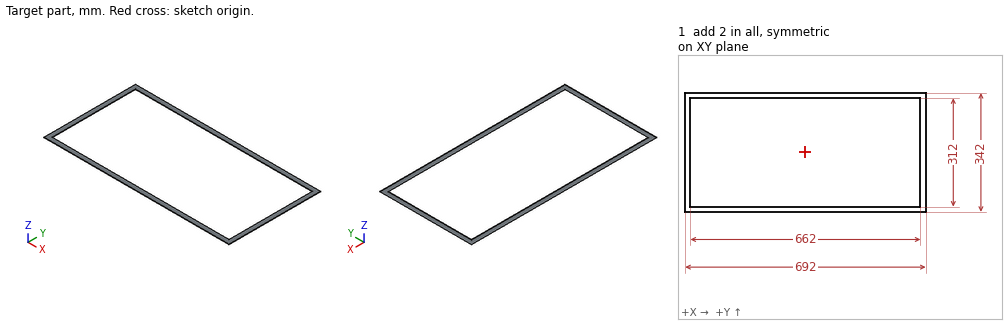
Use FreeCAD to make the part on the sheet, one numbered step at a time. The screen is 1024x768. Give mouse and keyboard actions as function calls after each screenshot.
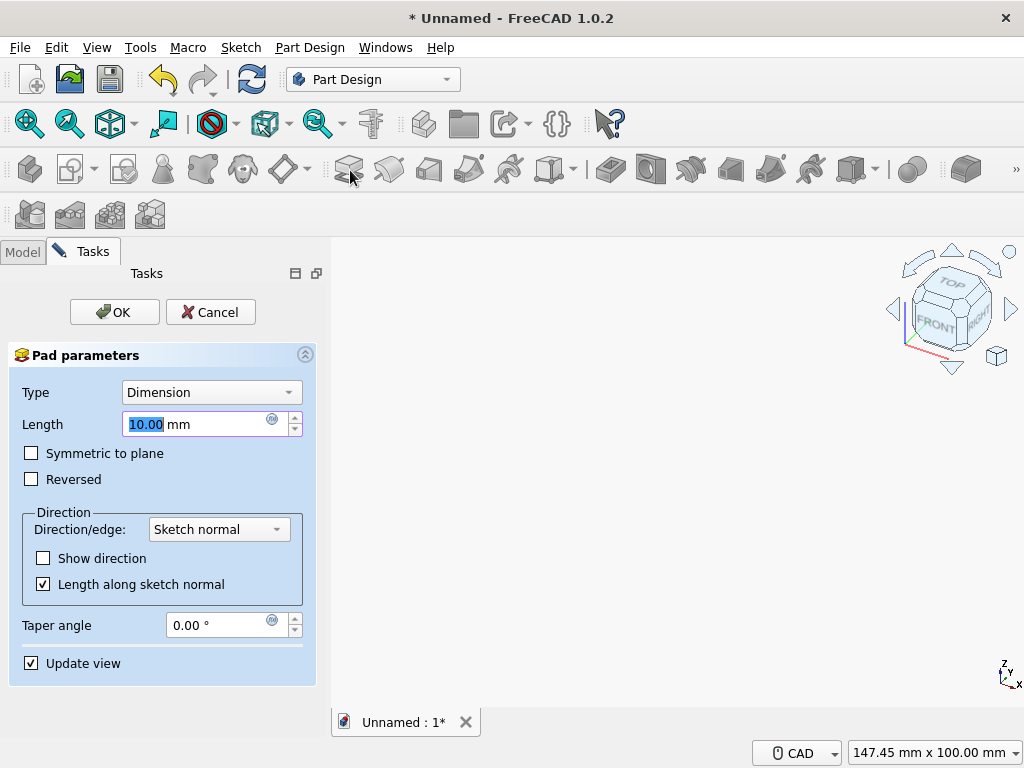
text(2)
key(Tab)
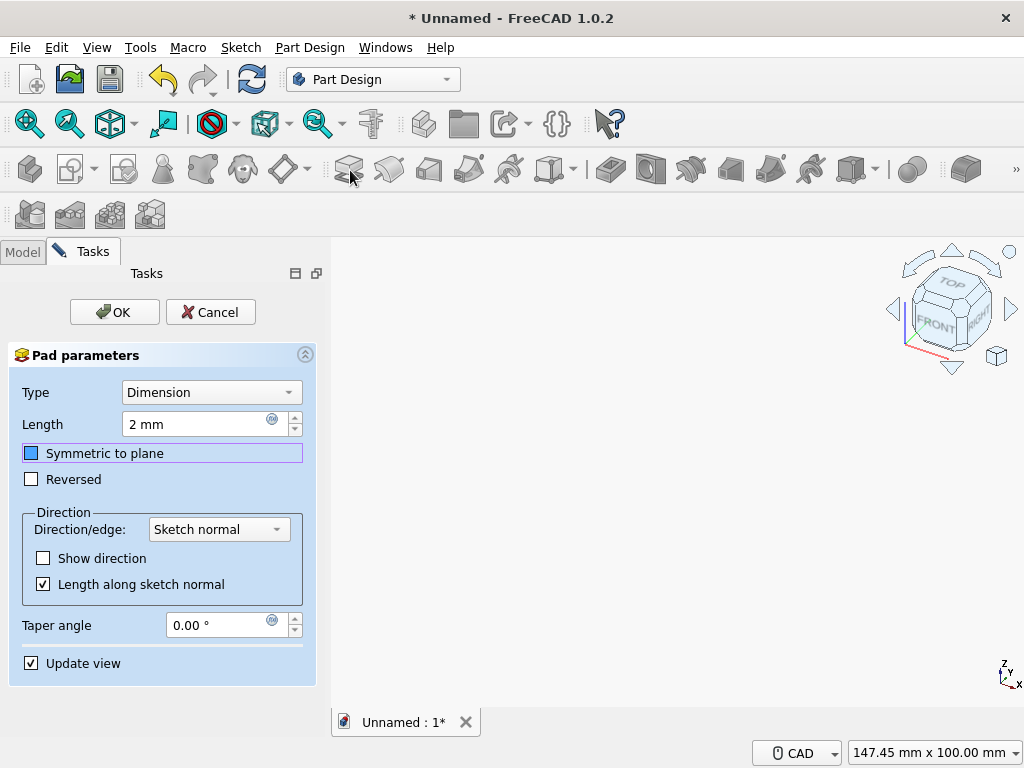
click(30, 453)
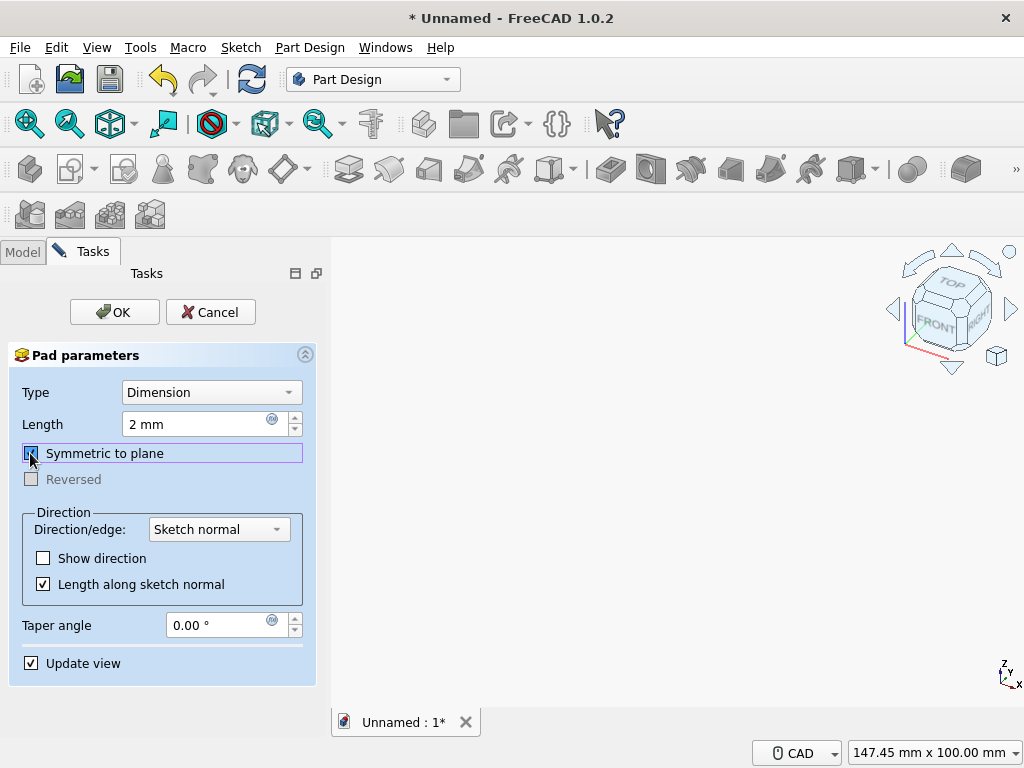
click(115, 312)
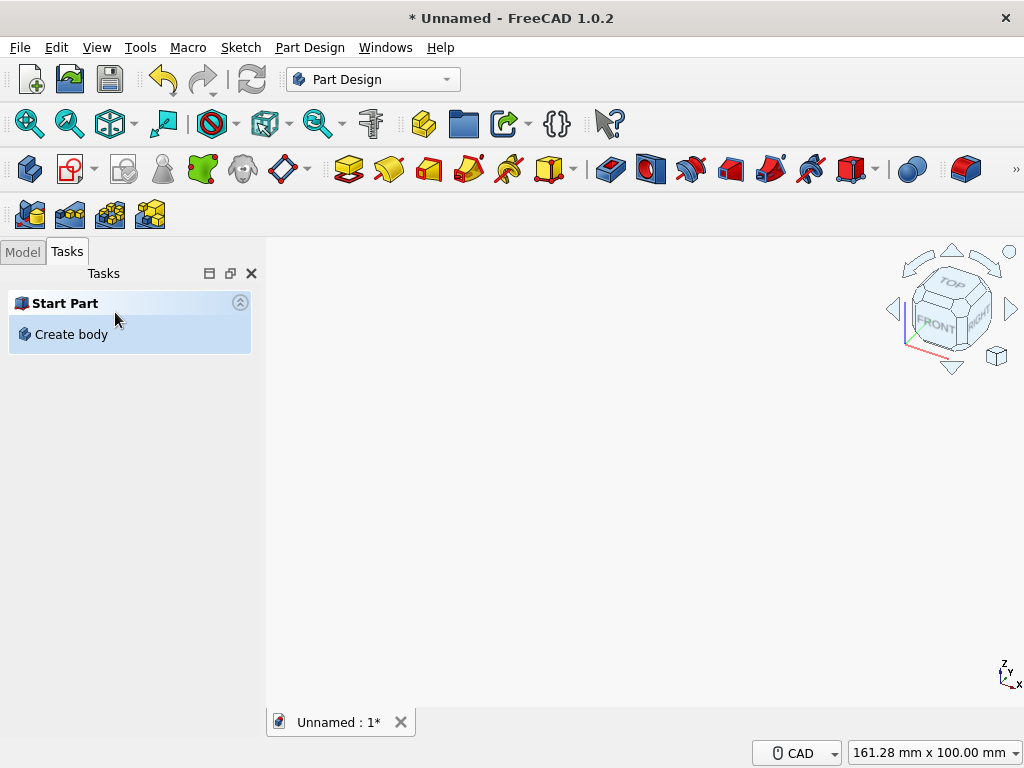
key(0)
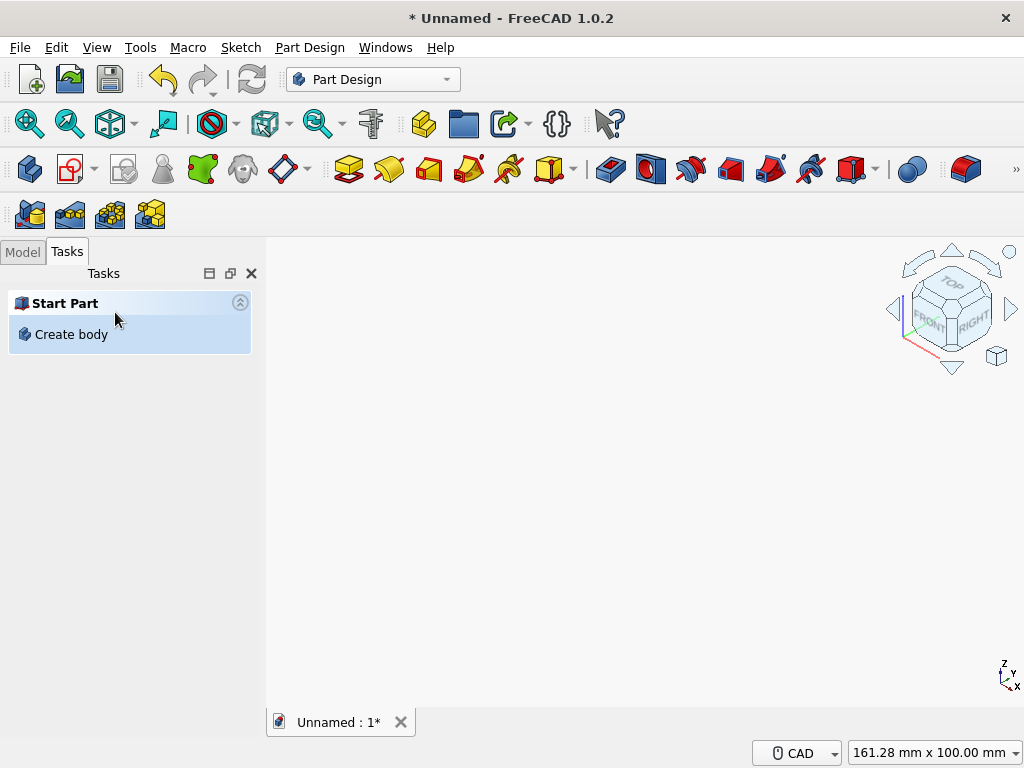
click(30, 124)